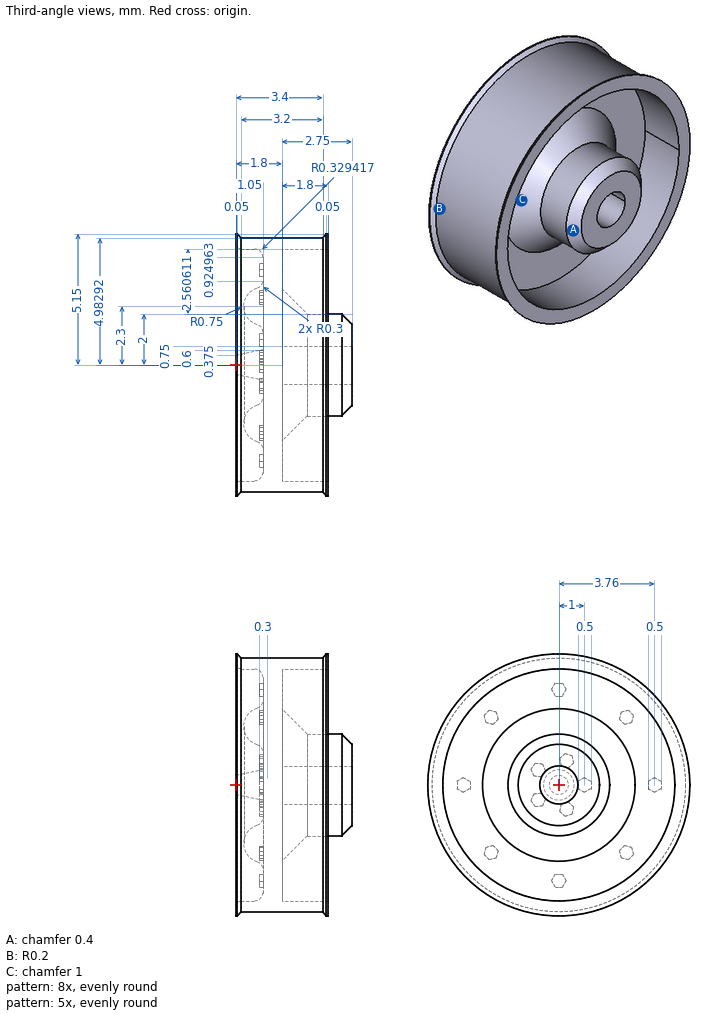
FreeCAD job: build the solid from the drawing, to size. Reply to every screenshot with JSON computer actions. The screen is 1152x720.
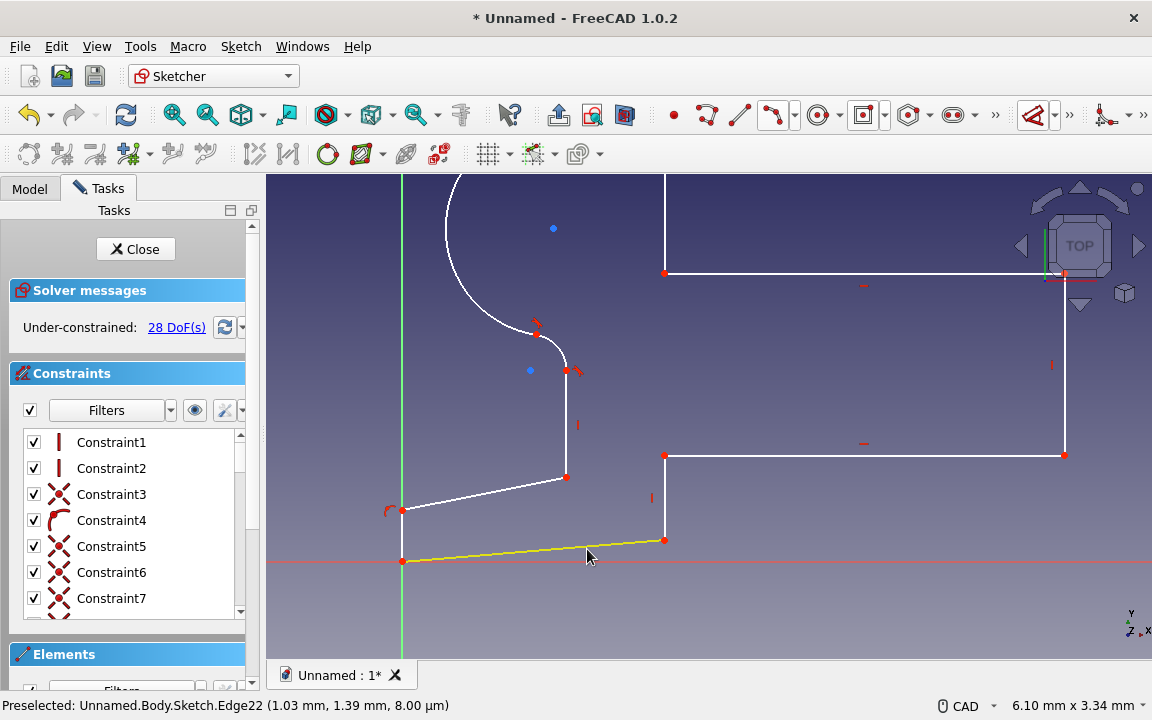
{"action": "left_click", "coordinate": [586, 547]}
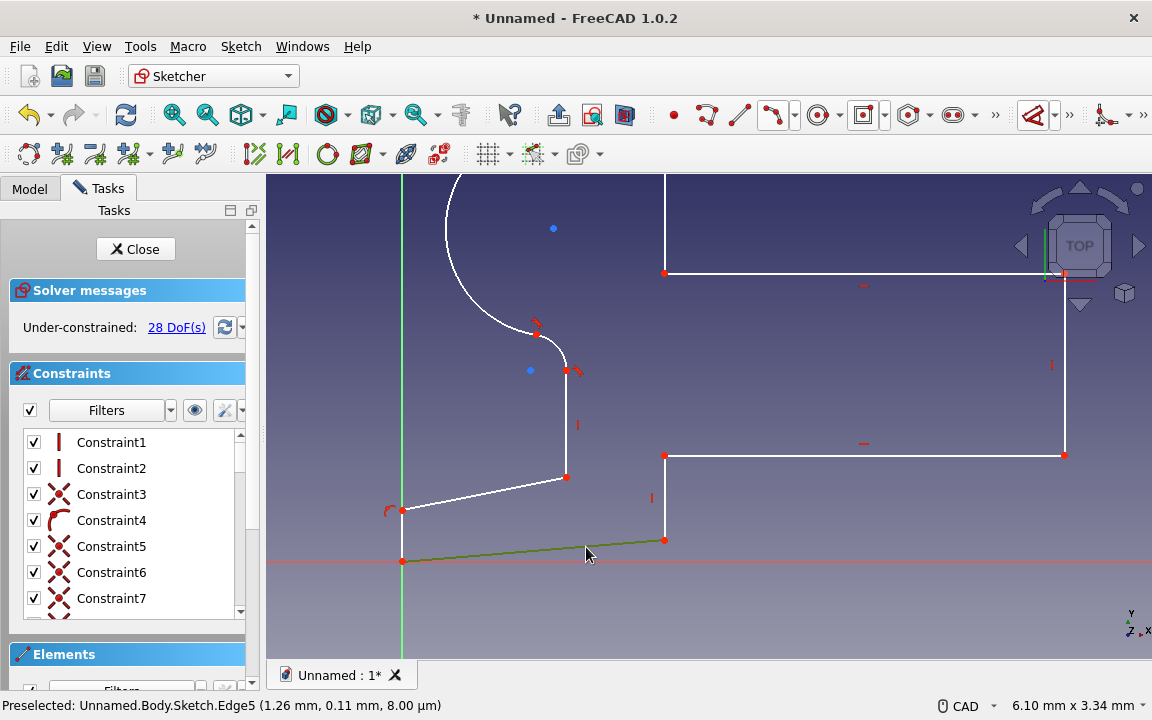
{"action": "key", "text": "h"}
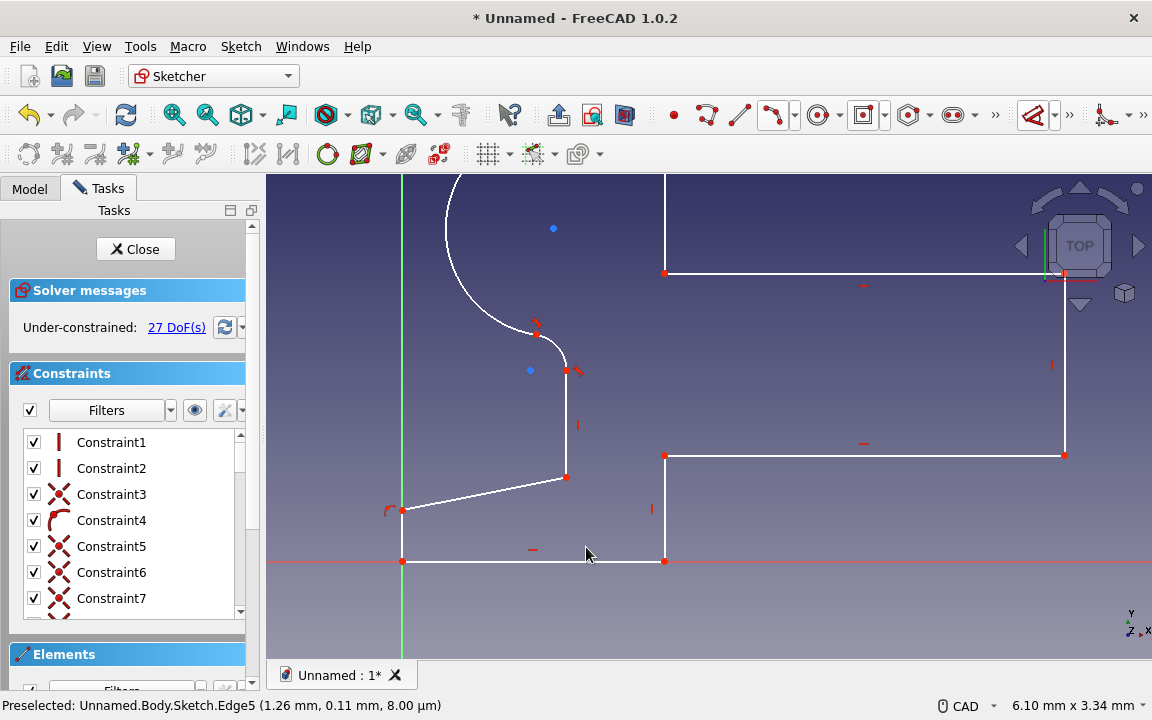
{"action": "scroll", "coordinate": [587, 550], "scroll_direction": "down", "scroll_amount": 5}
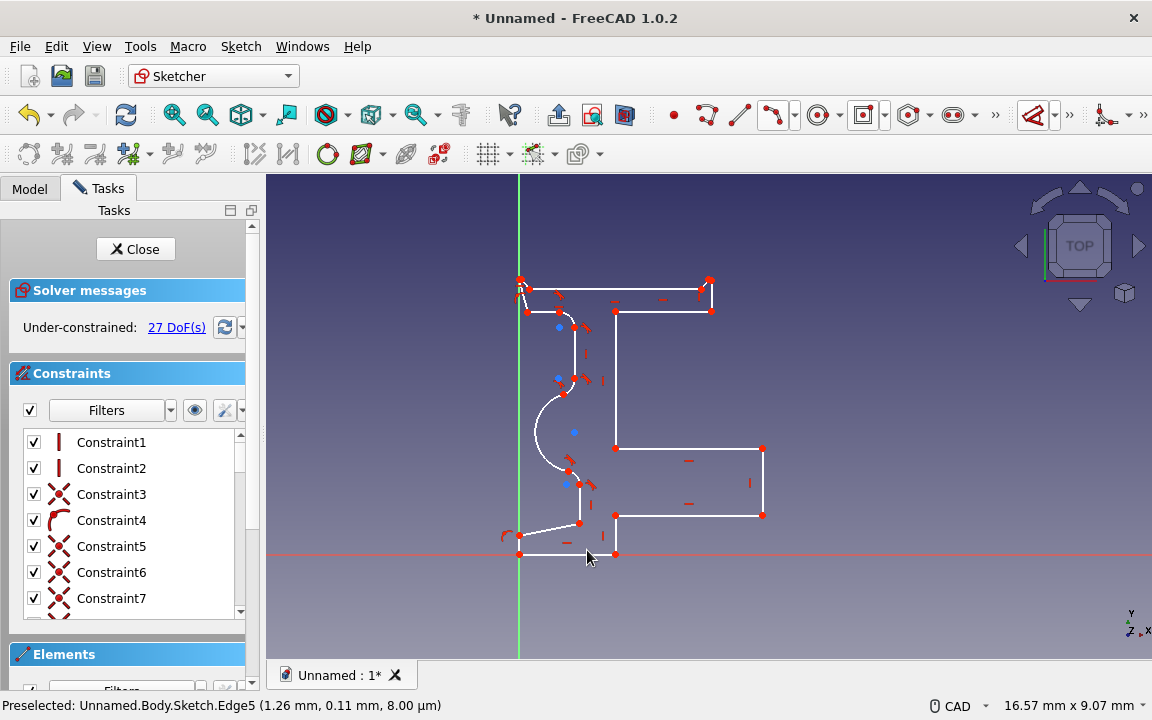
{"action": "scroll", "coordinate": [710, 280], "scroll_direction": "up", "scroll_amount": 12}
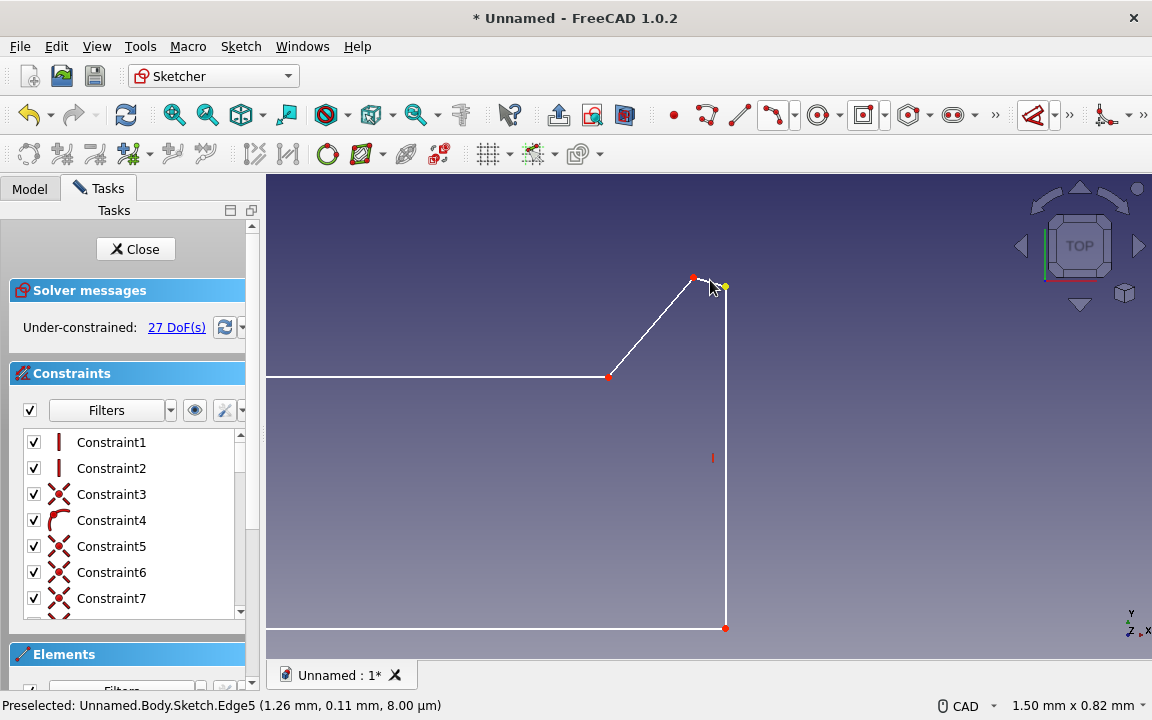
{"action": "left_click", "coordinate": [710, 282]}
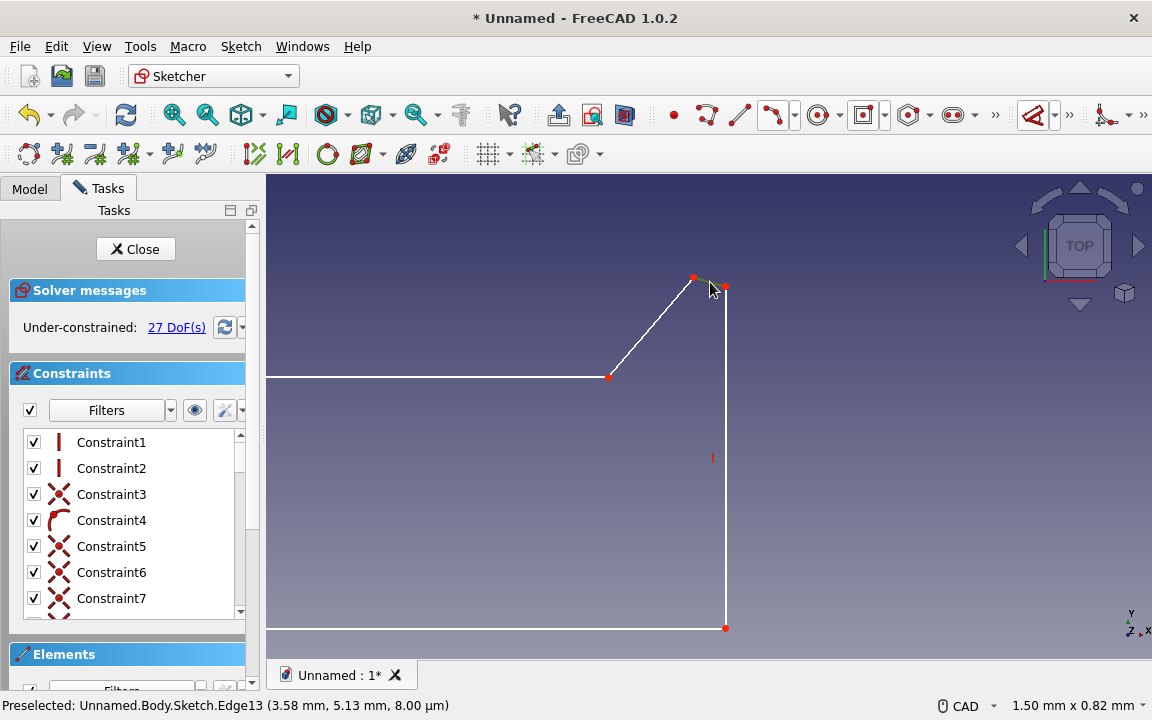
{"action": "key", "text": "h"}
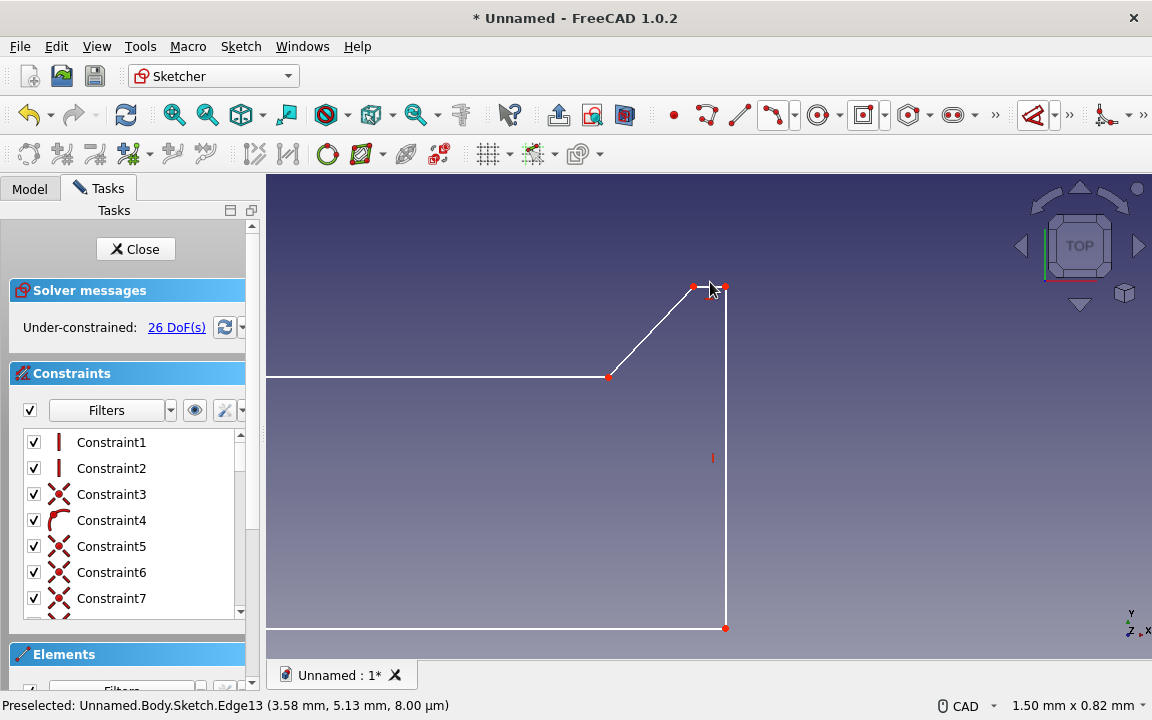
{"action": "scroll", "coordinate": [710, 279], "scroll_direction": "down", "scroll_amount": 12}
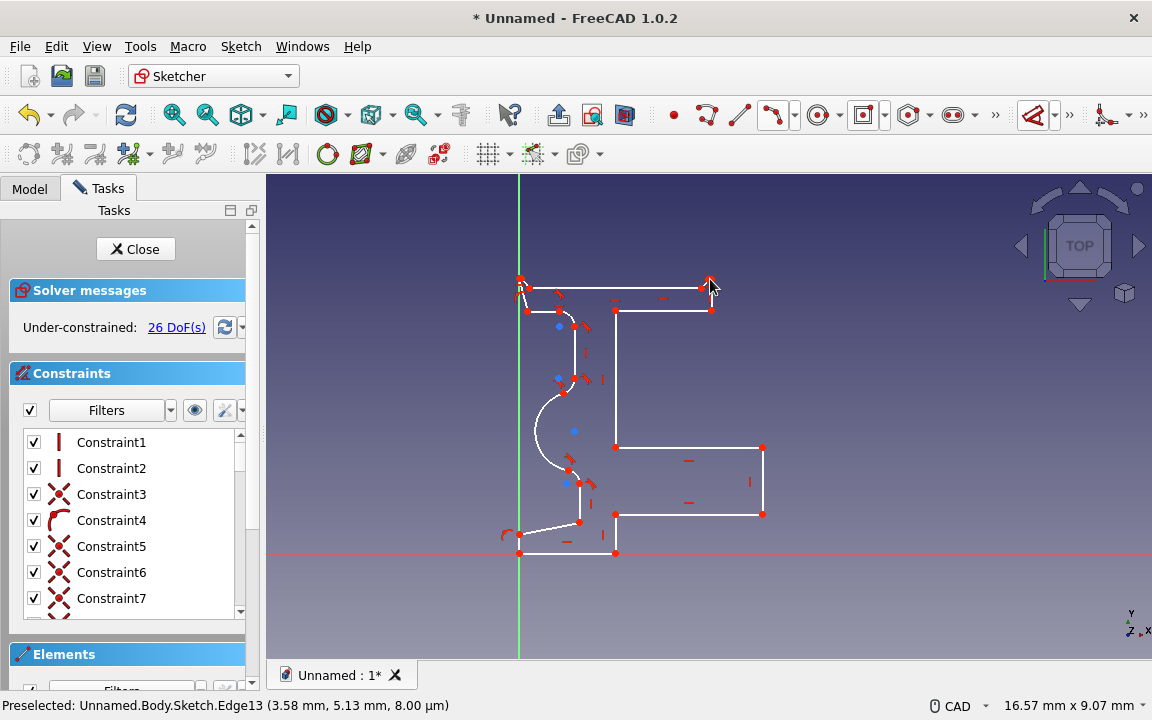
{"action": "scroll", "coordinate": [522, 289], "scroll_direction": "up", "scroll_amount": 9}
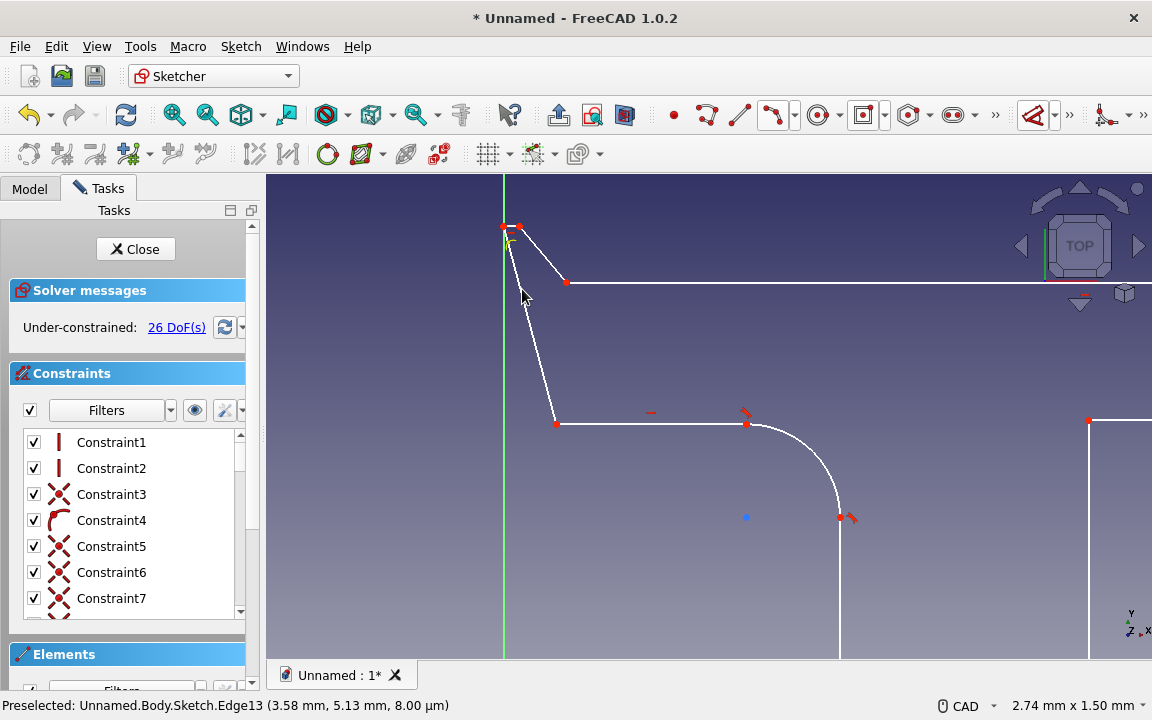
{"action": "left_click", "coordinate": [520, 286]}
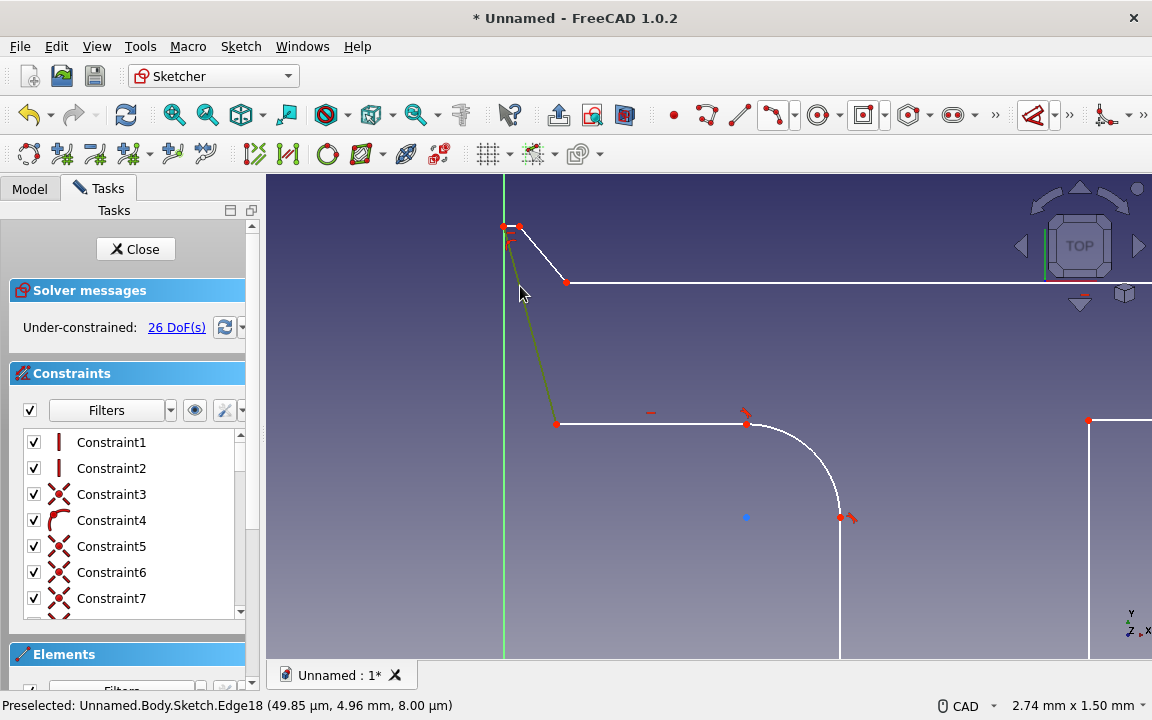
{"action": "key", "text": "v"}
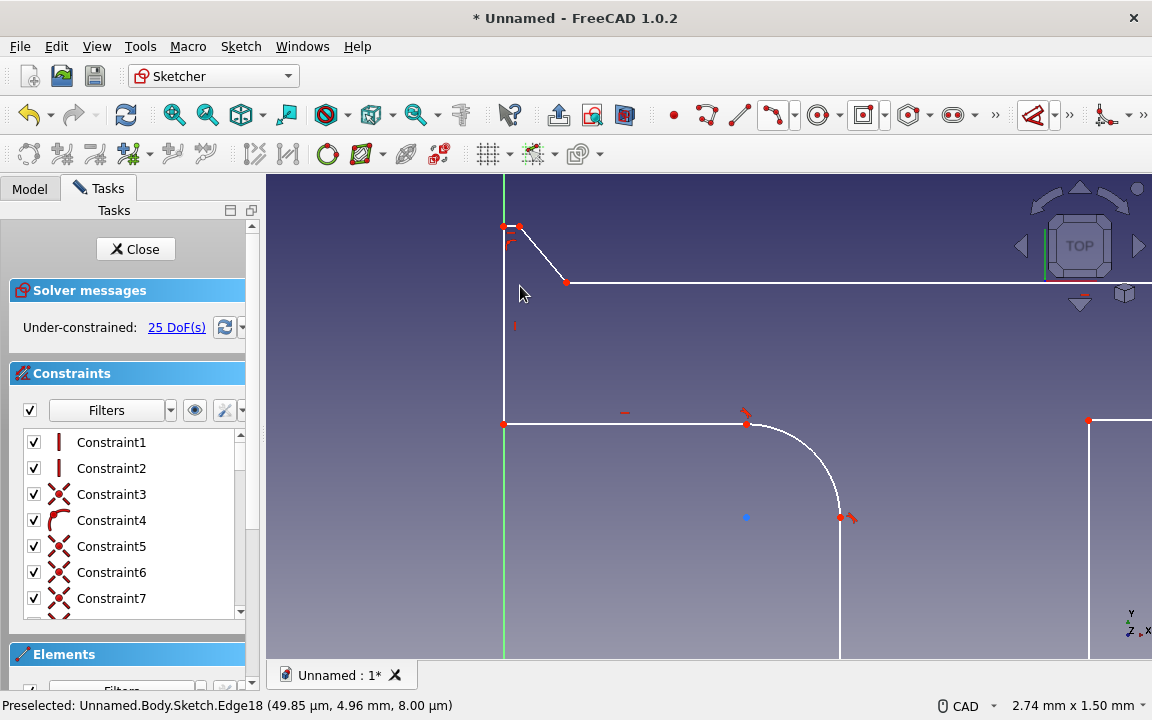
{"action": "scroll", "coordinate": [522, 289], "scroll_direction": "down", "scroll_amount": 9}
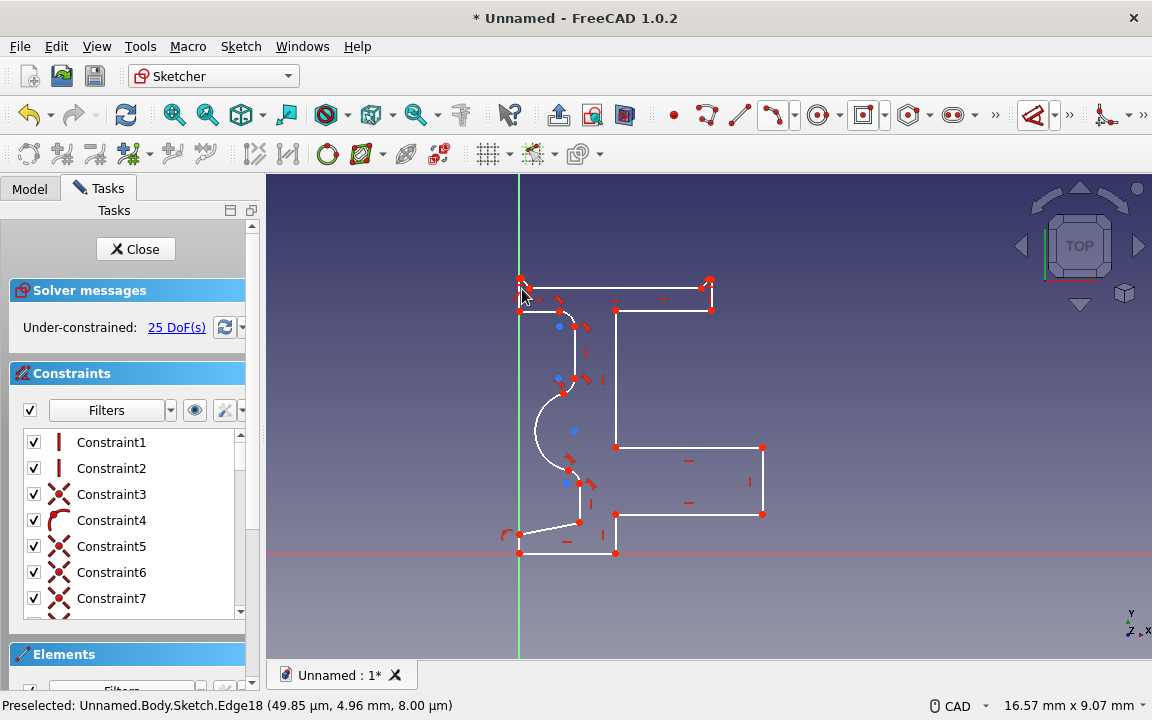
{"action": "scroll", "coordinate": [569, 391], "scroll_direction": "up", "scroll_amount": 4}